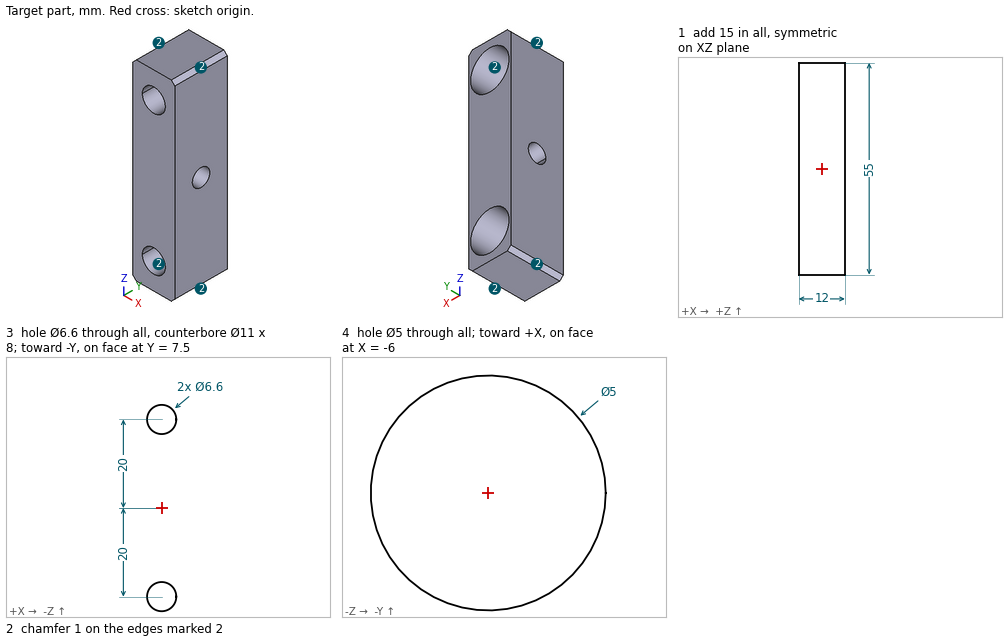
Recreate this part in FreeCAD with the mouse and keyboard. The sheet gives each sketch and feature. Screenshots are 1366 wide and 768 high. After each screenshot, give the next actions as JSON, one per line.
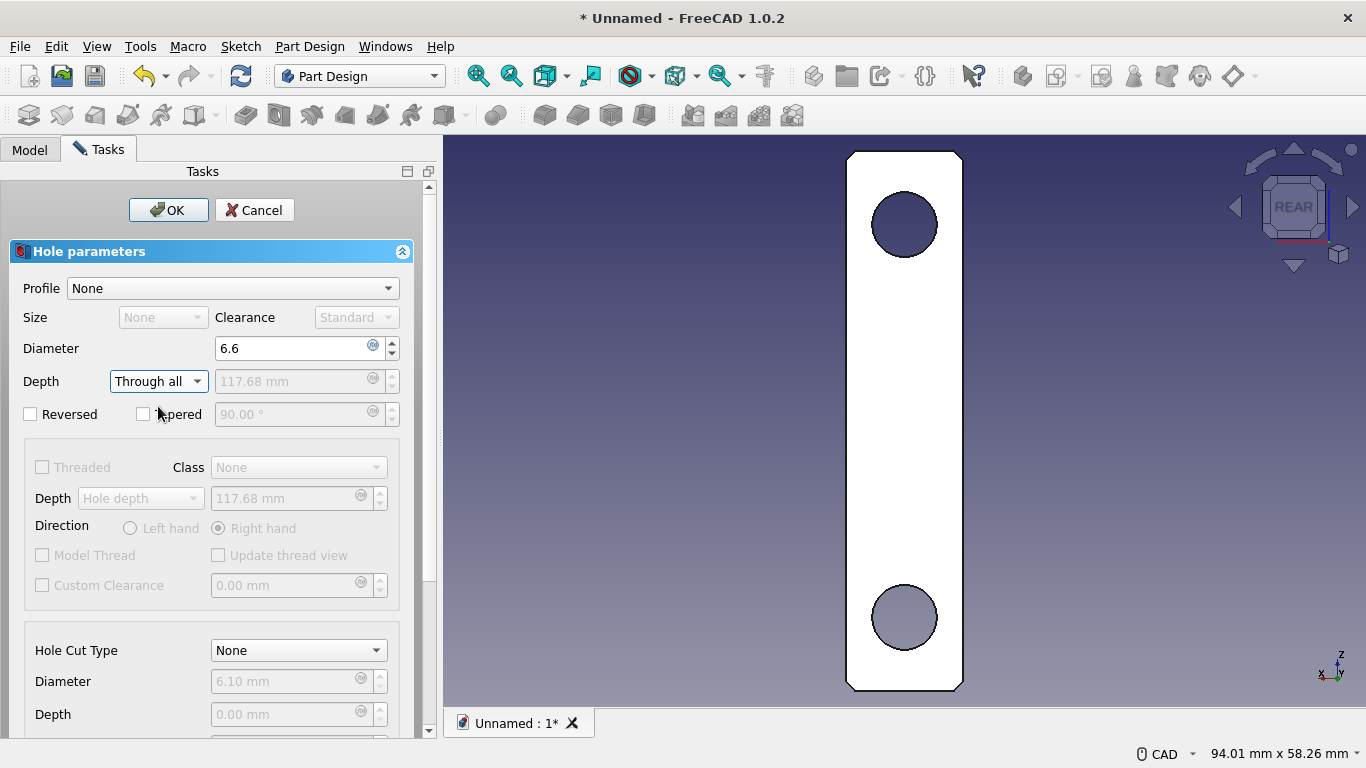
{"action": "left_click", "coordinate": [300, 650]}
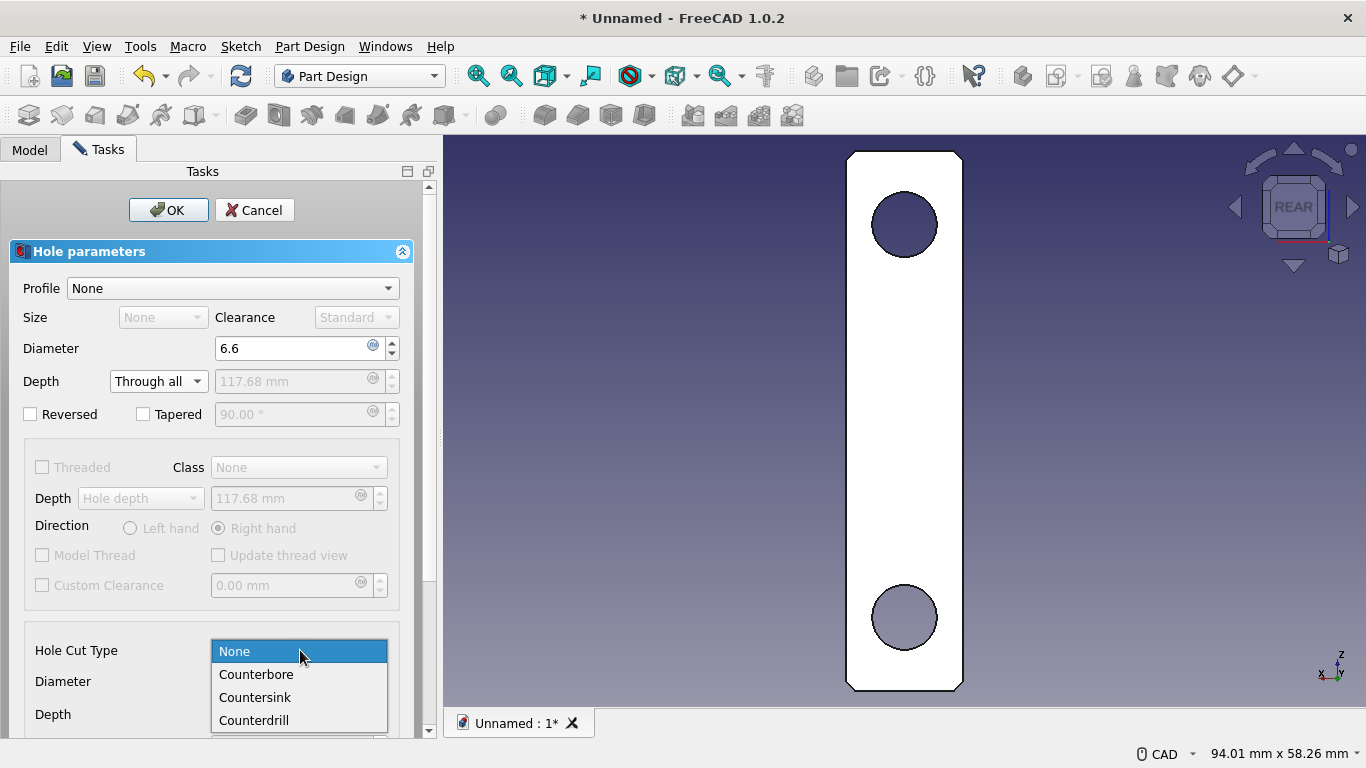
{"action": "left_click", "coordinate": [298, 674]}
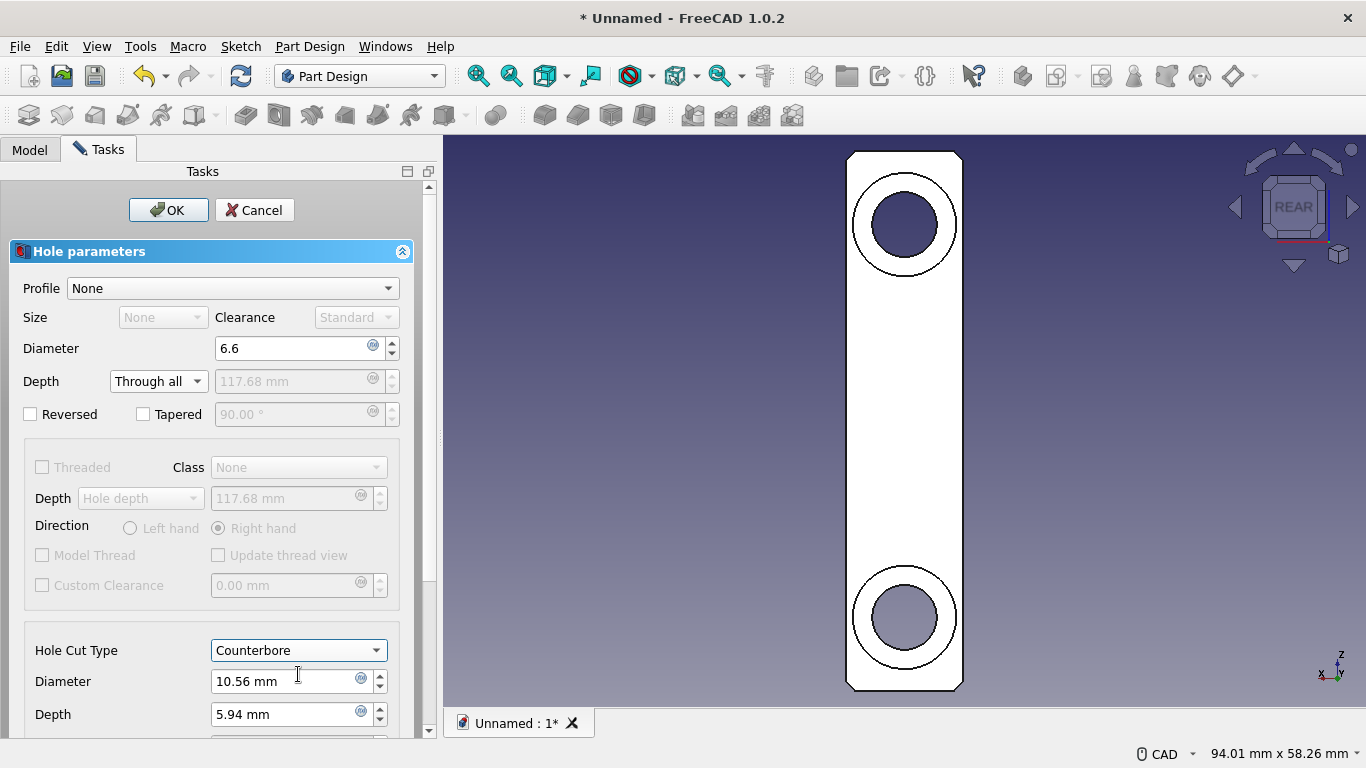
{"action": "triple_click", "coordinate": [292, 682]}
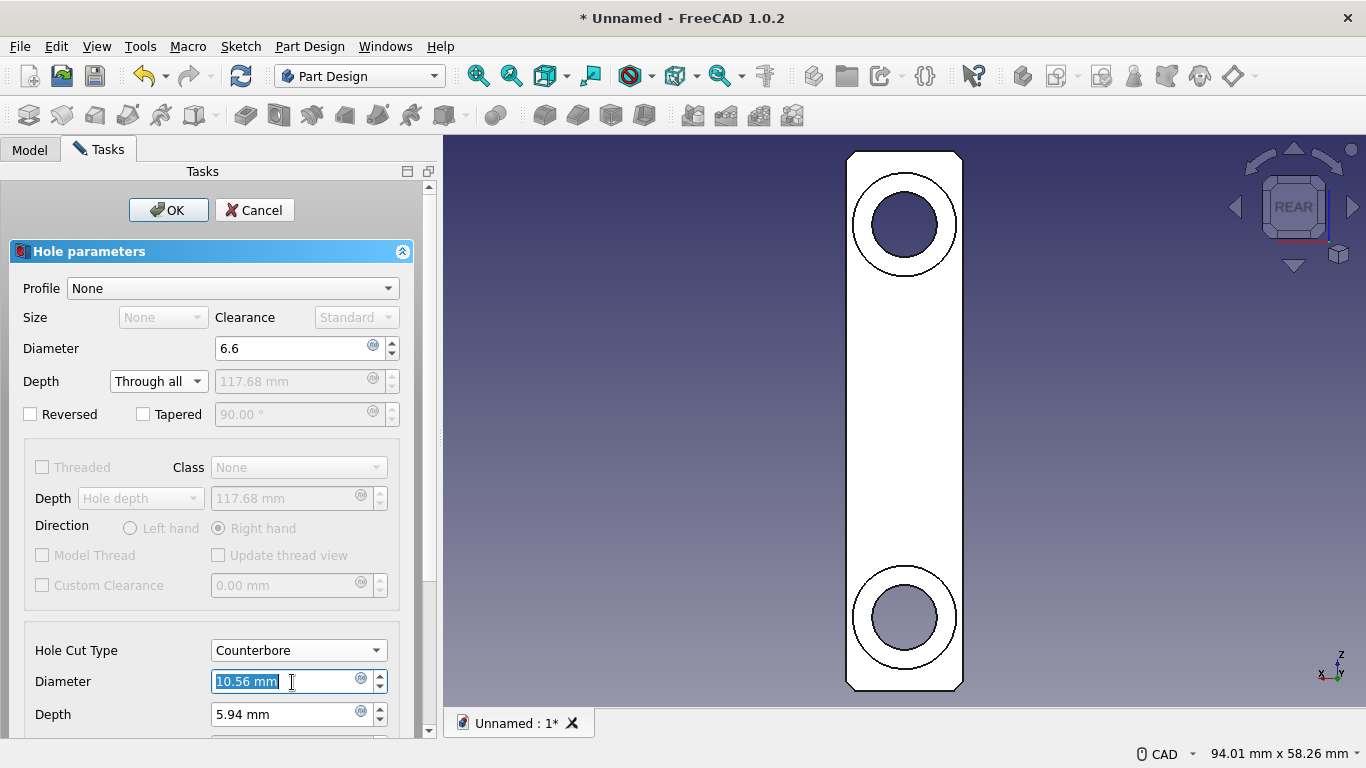
{"action": "type", "text": "11"}
{"action": "key", "text": "Tab"}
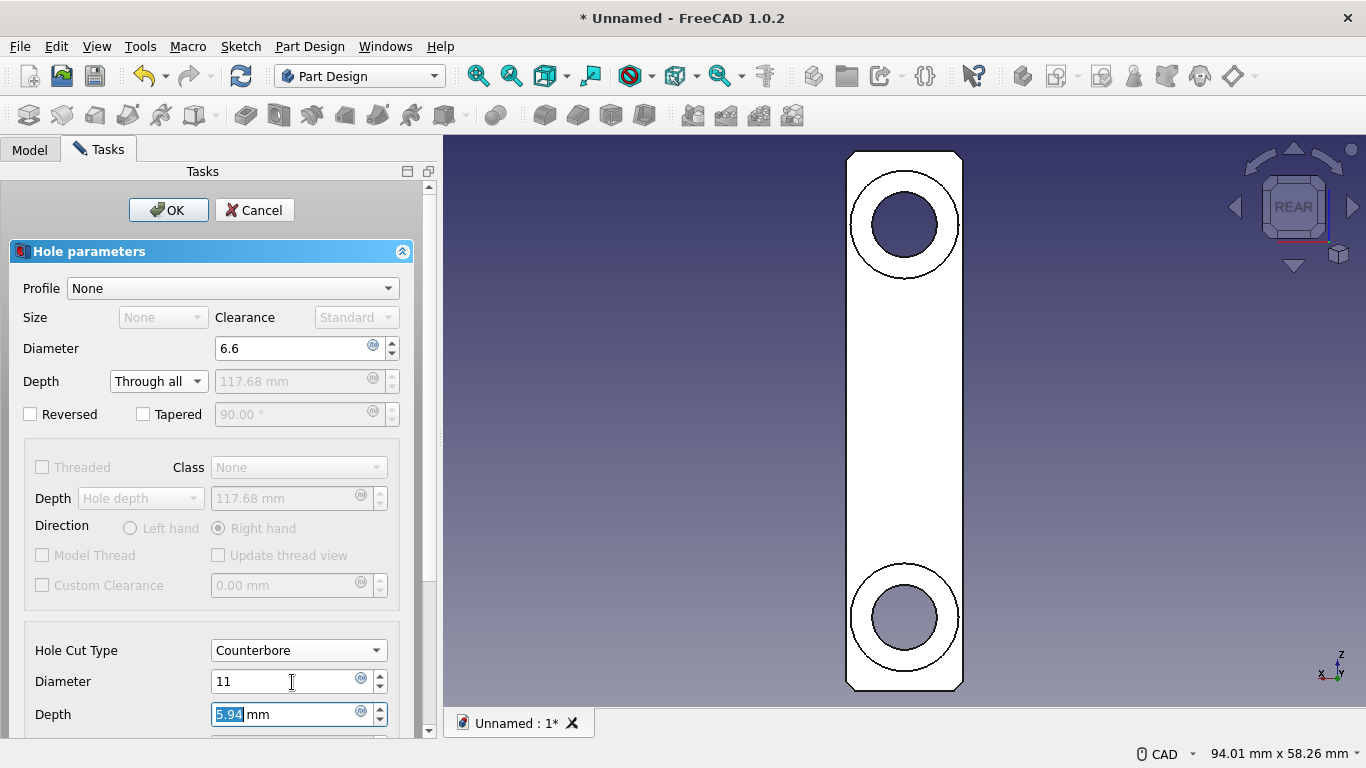
{"action": "type", "text": "8"}
{"action": "key", "text": "Tab"}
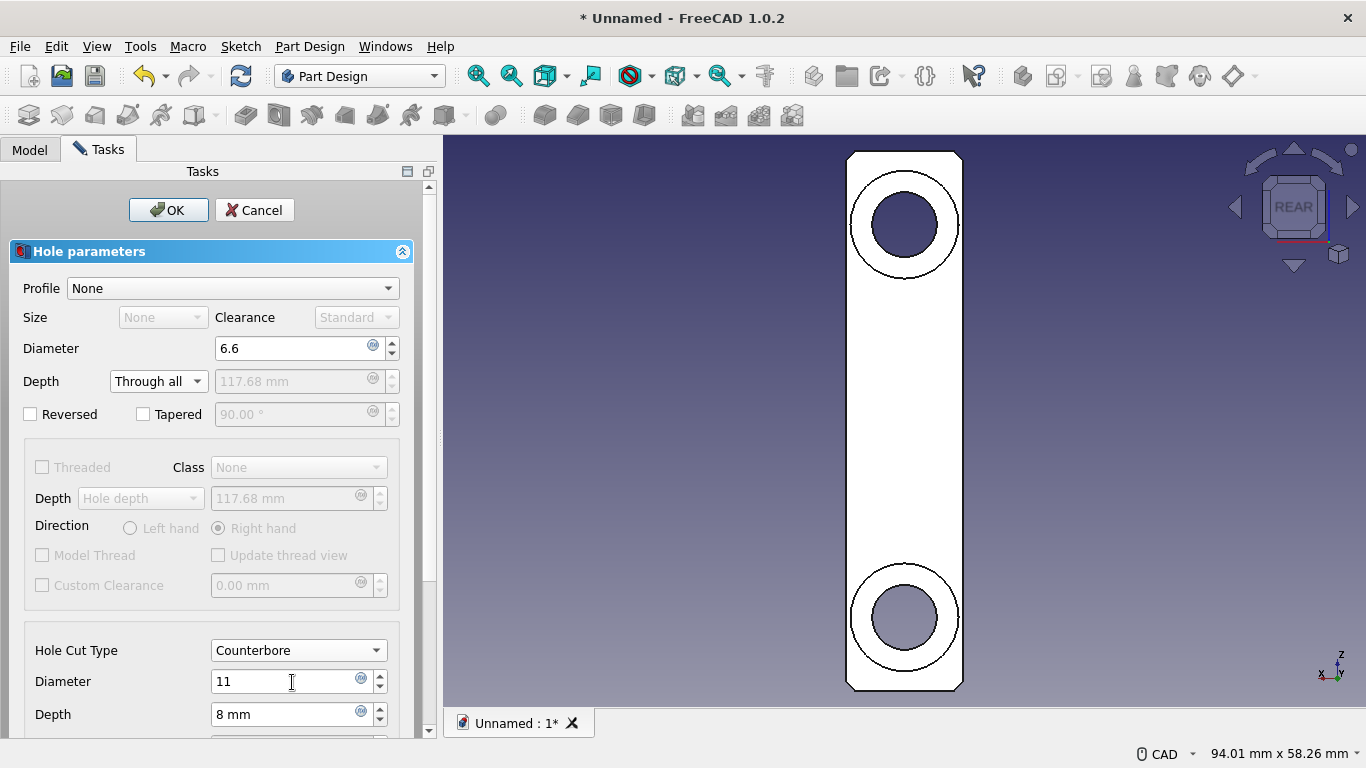
{"action": "left_click", "coordinate": [169, 210]}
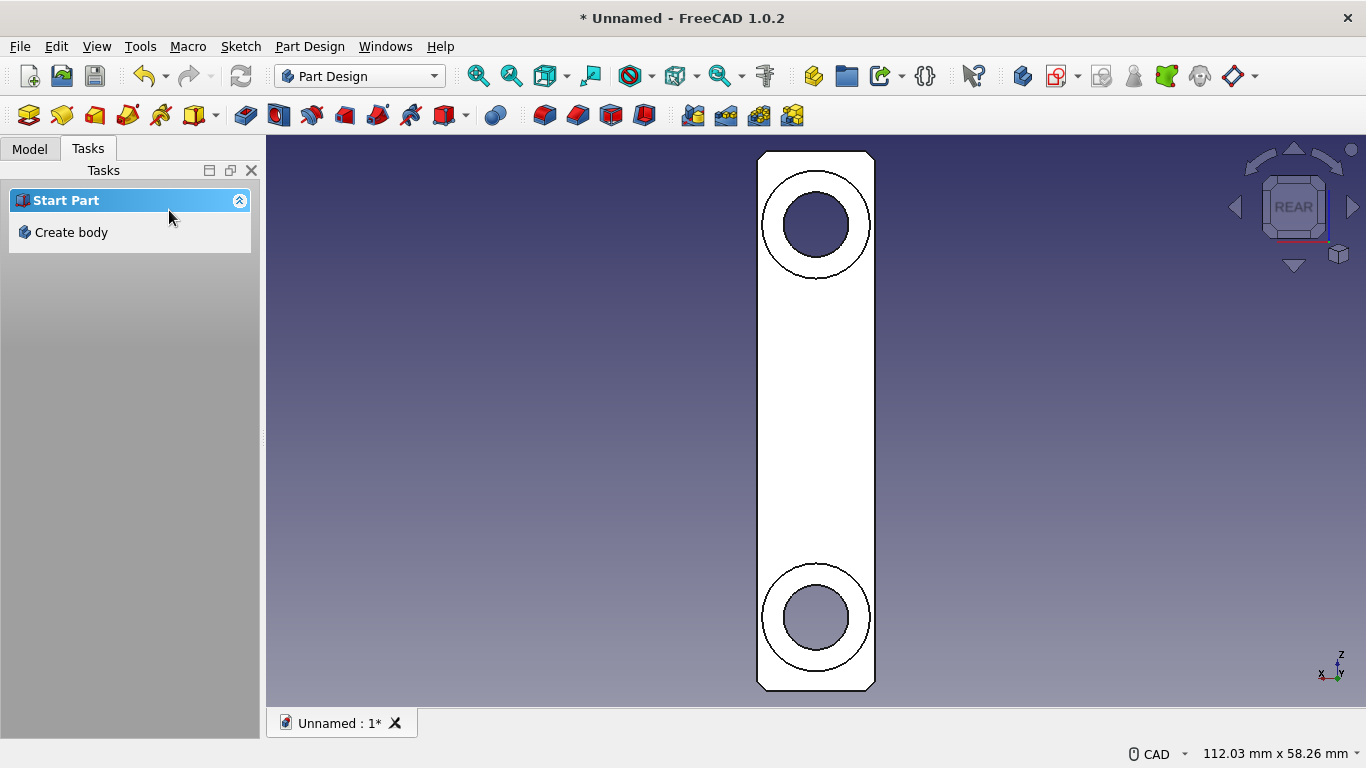
{"action": "key", "text": "6"}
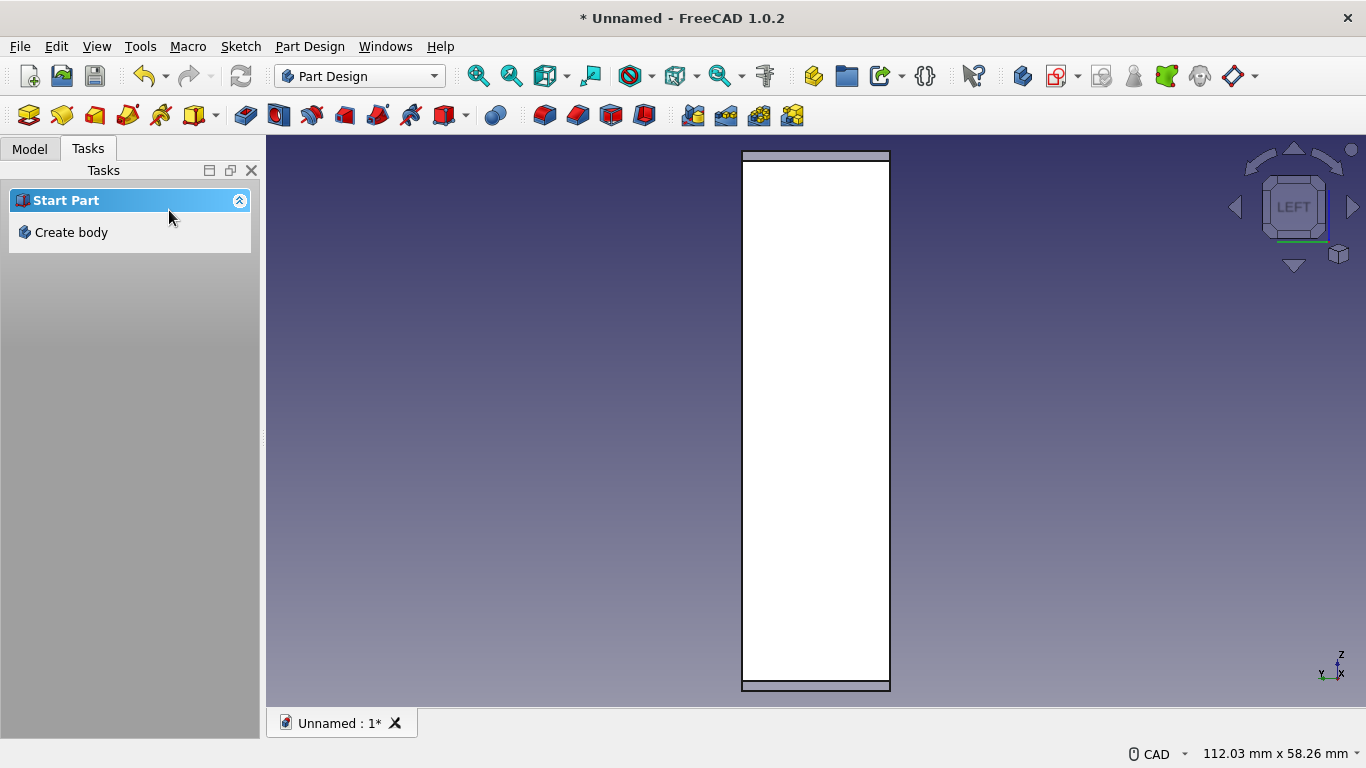
{"action": "left_click", "coordinate": [816, 271]}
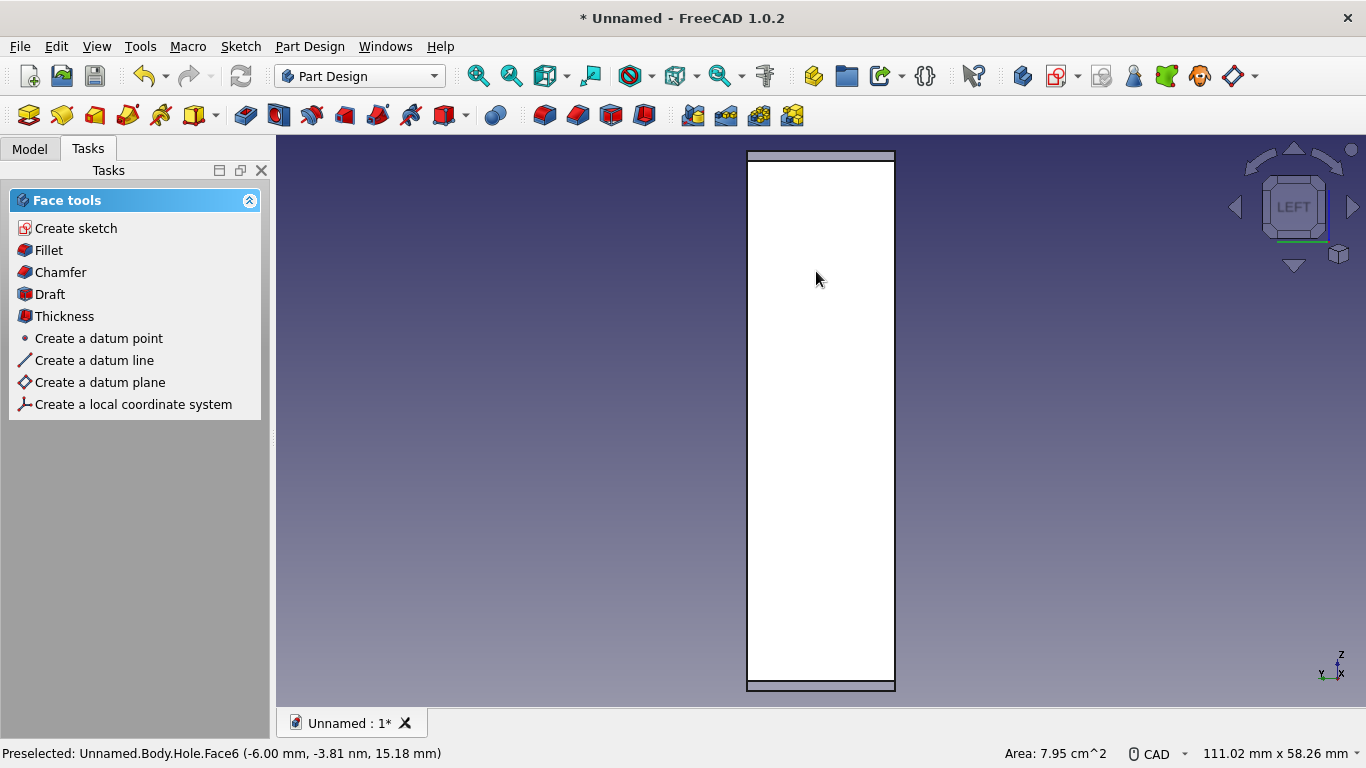
{"action": "left_click", "coordinate": [1056, 76]}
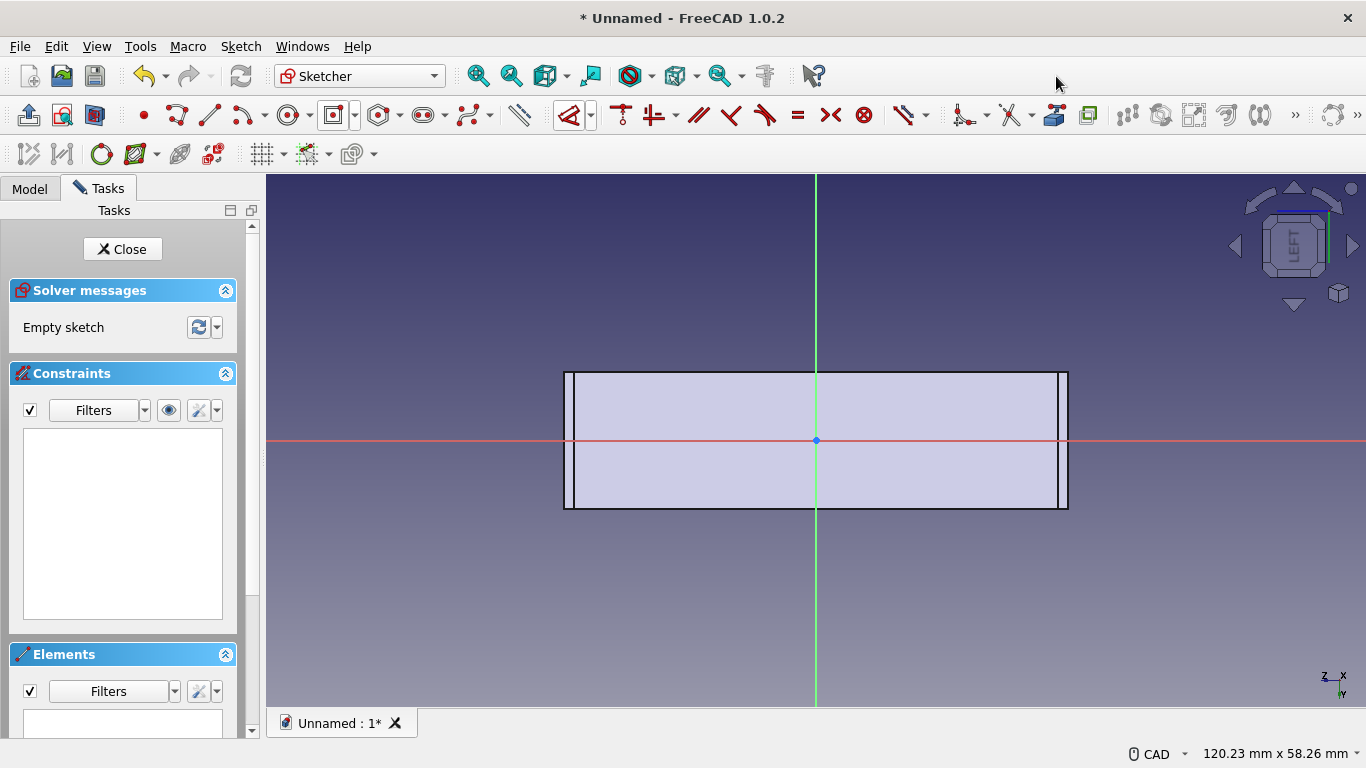
{"action": "scroll", "coordinate": [827, 441], "scroll_direction": "up", "scroll_amount": 10}